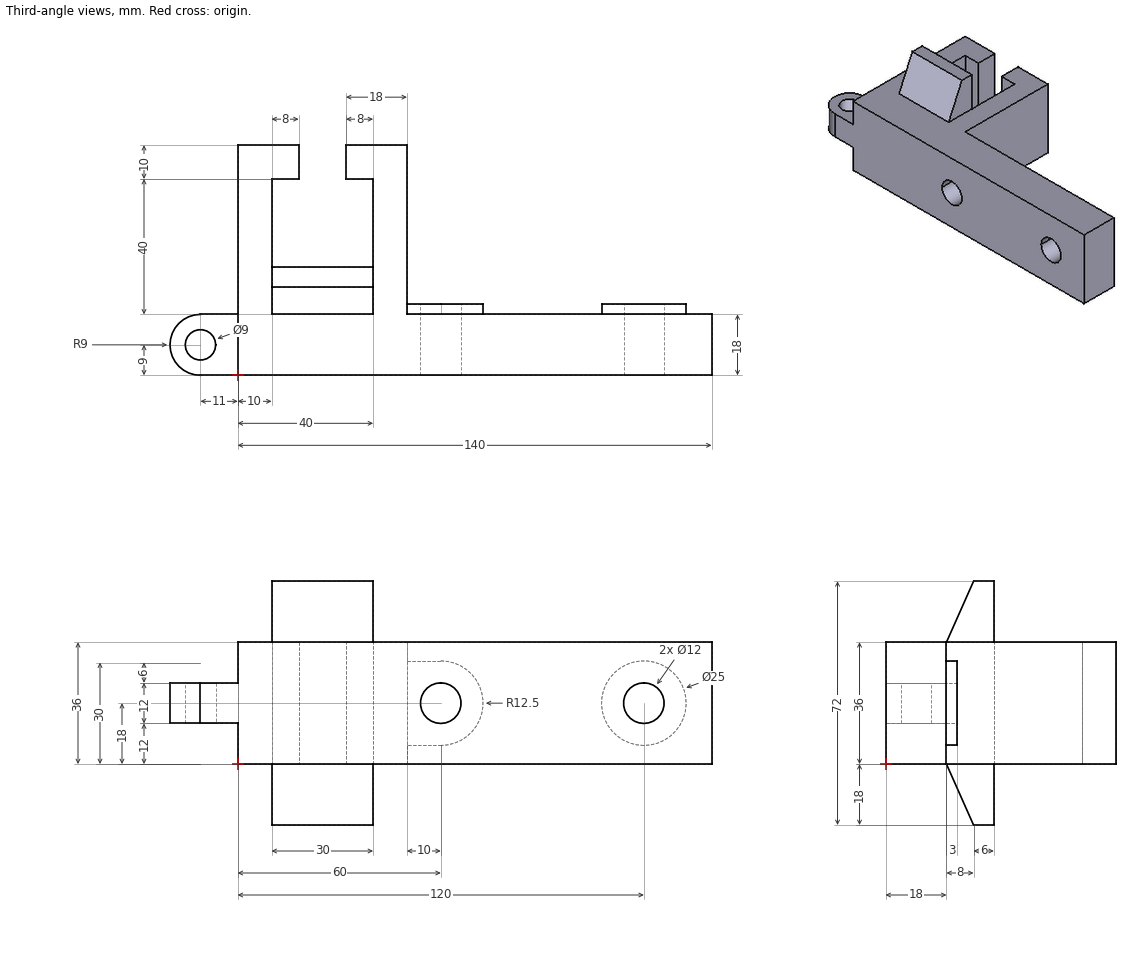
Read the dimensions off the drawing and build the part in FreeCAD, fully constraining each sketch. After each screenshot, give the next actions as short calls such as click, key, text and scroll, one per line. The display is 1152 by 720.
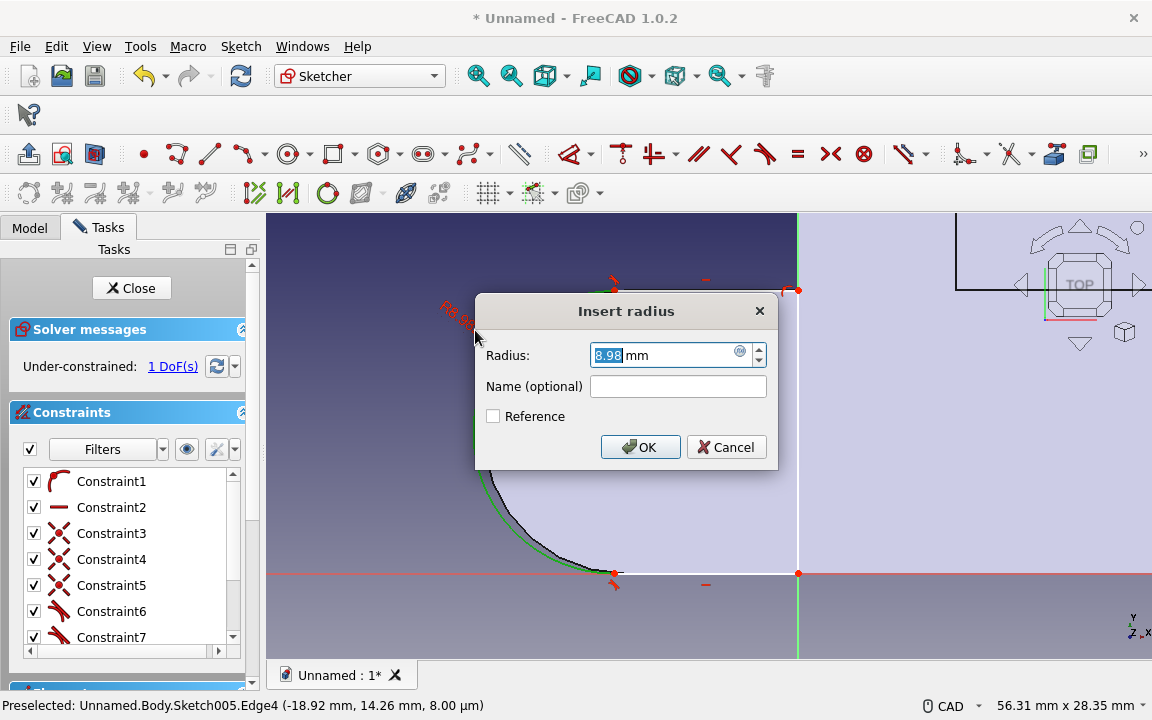
text(9)
key(Return)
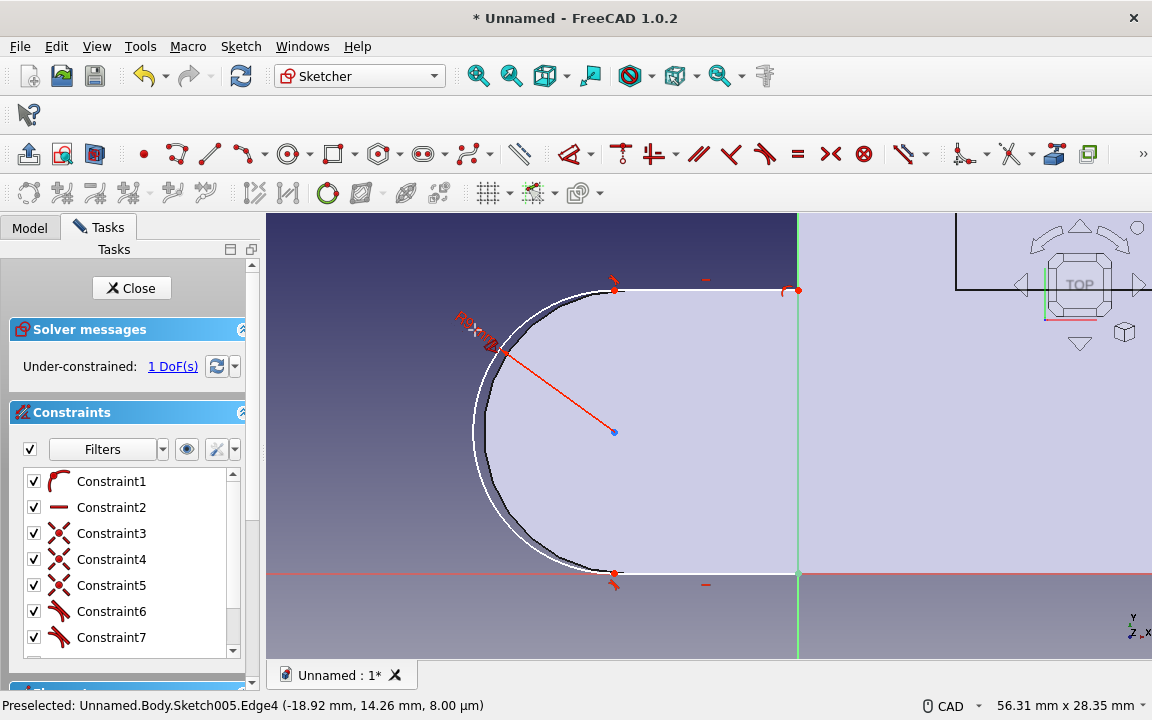
click(670, 290)
click(707, 256)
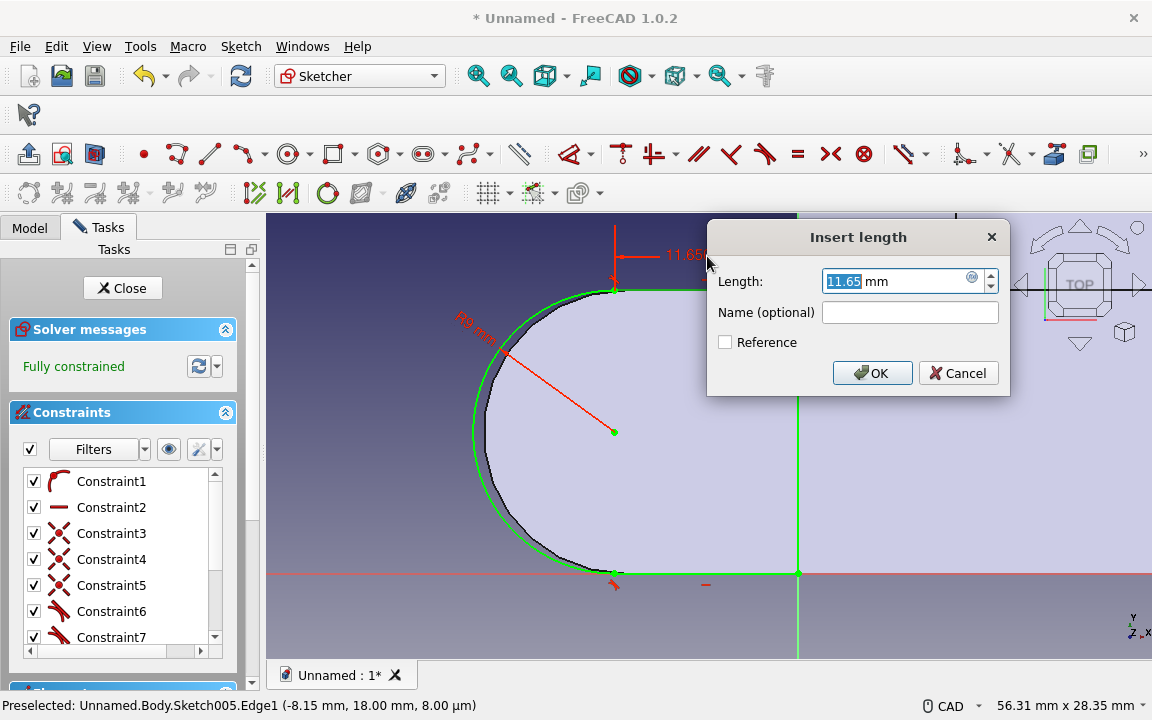
text(11)
key(Return)
key(Escape)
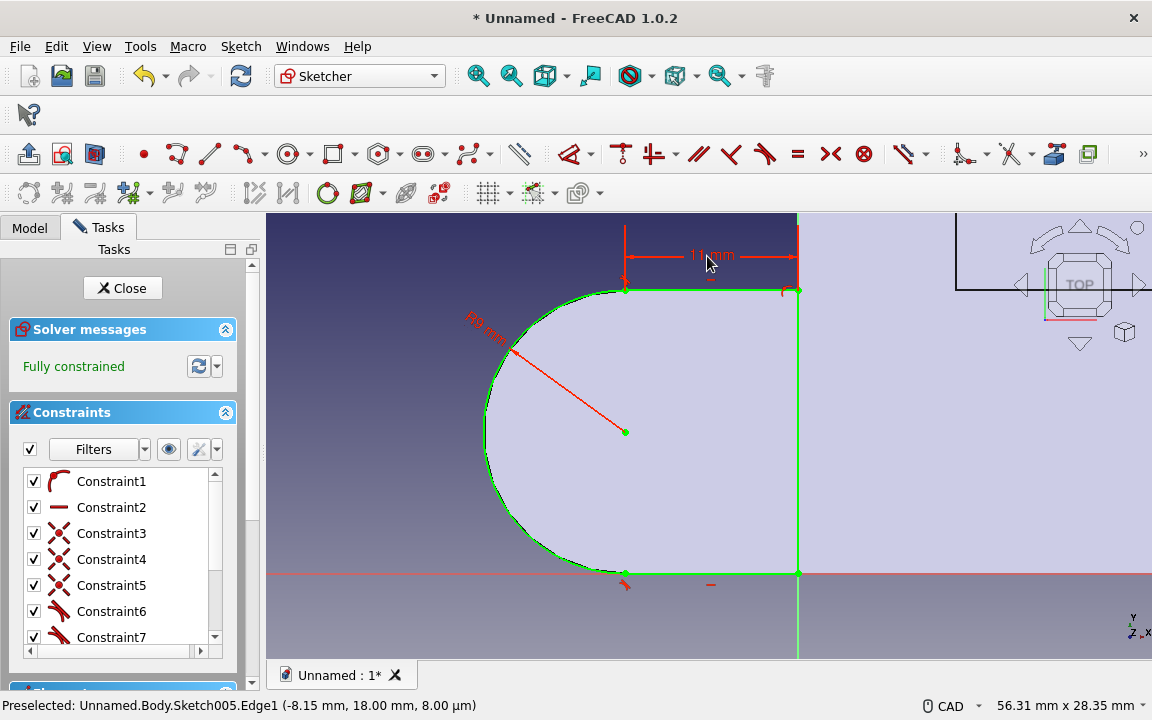
click(123, 288)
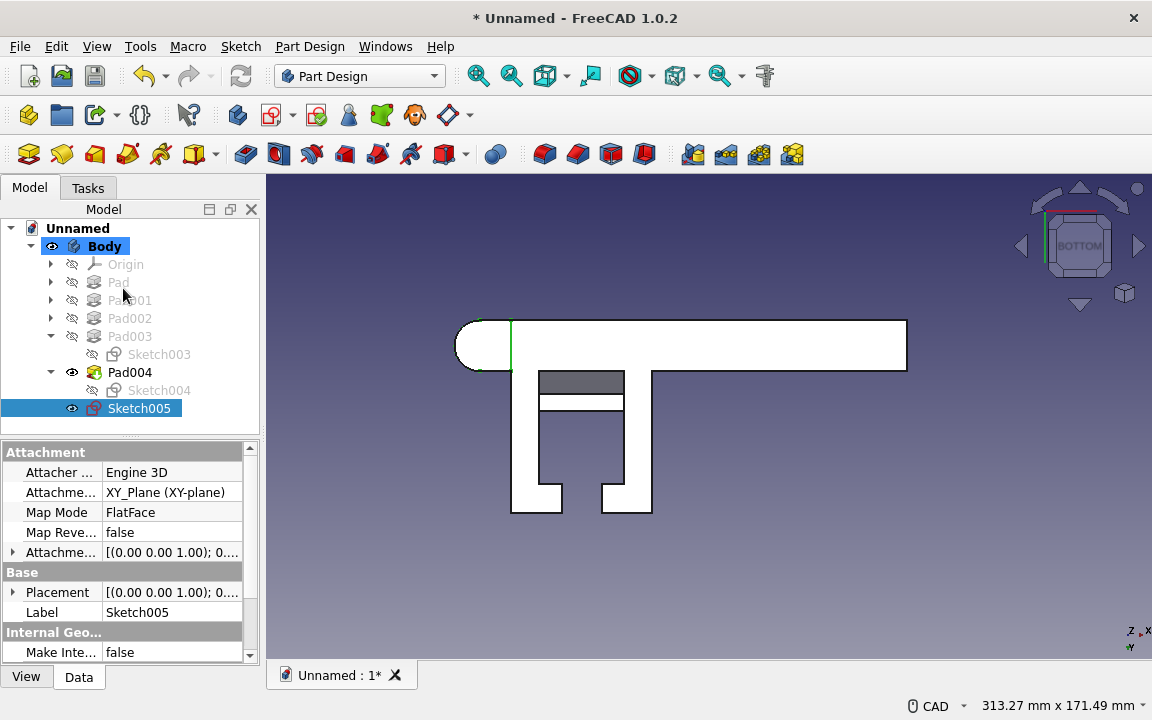
click(246, 154)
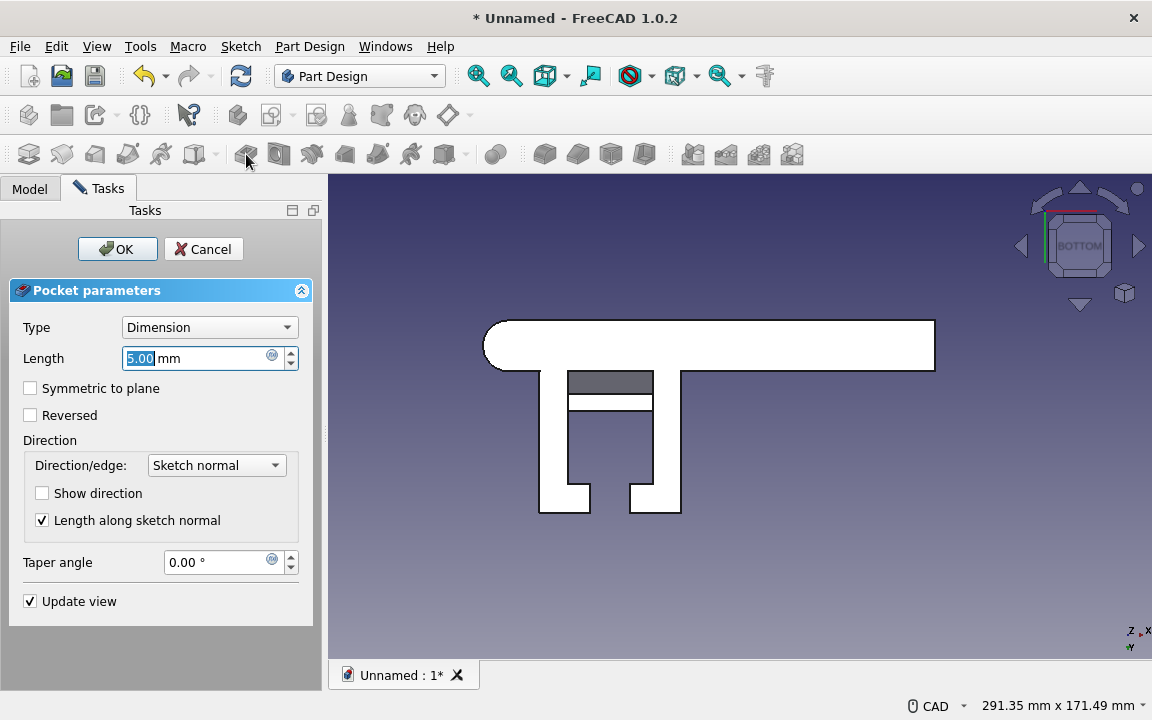
text(12)
key(Tab)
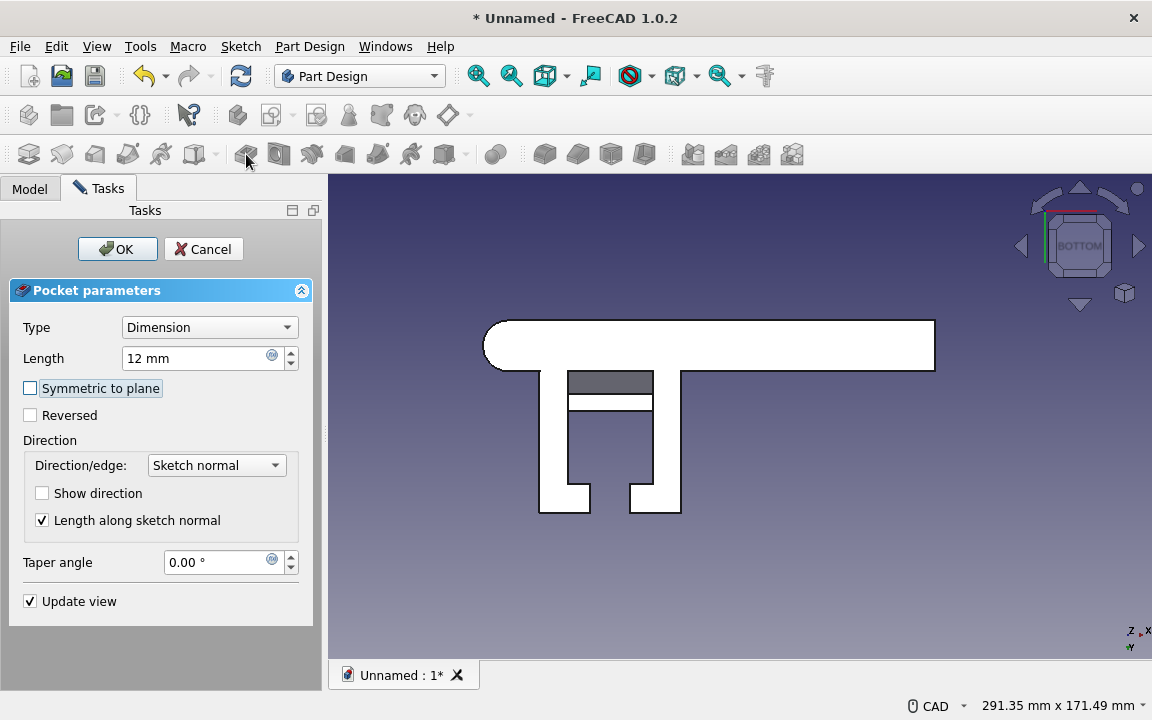
click(31, 415)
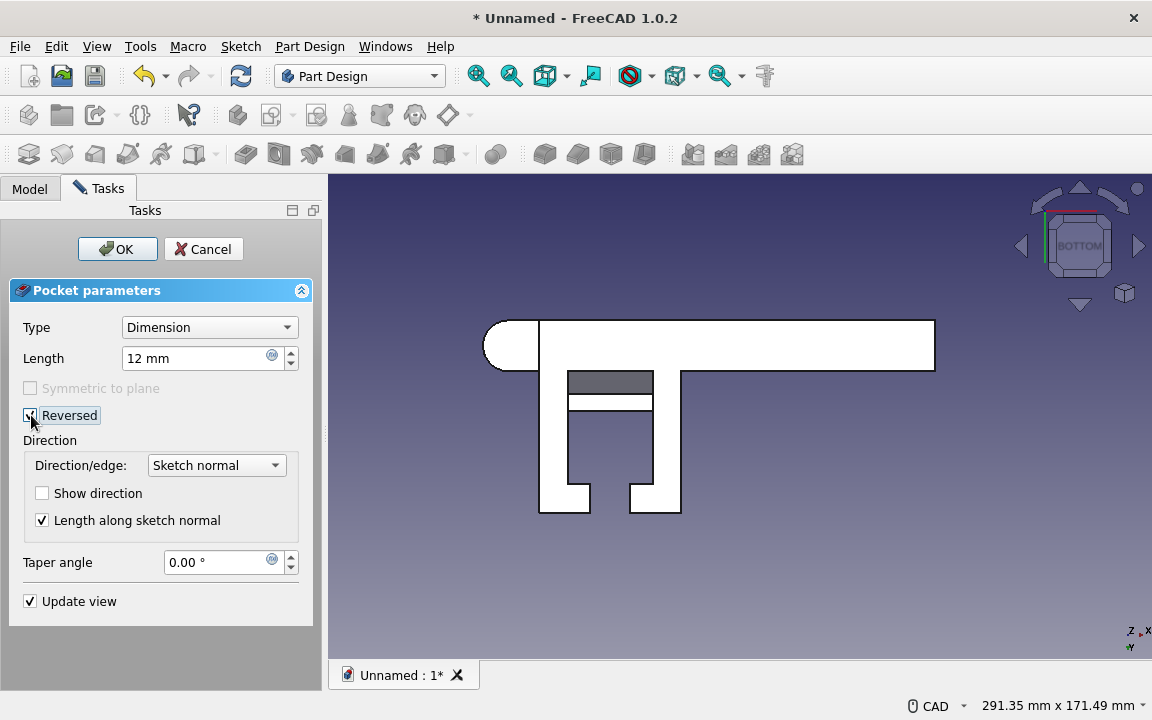
click(118, 249)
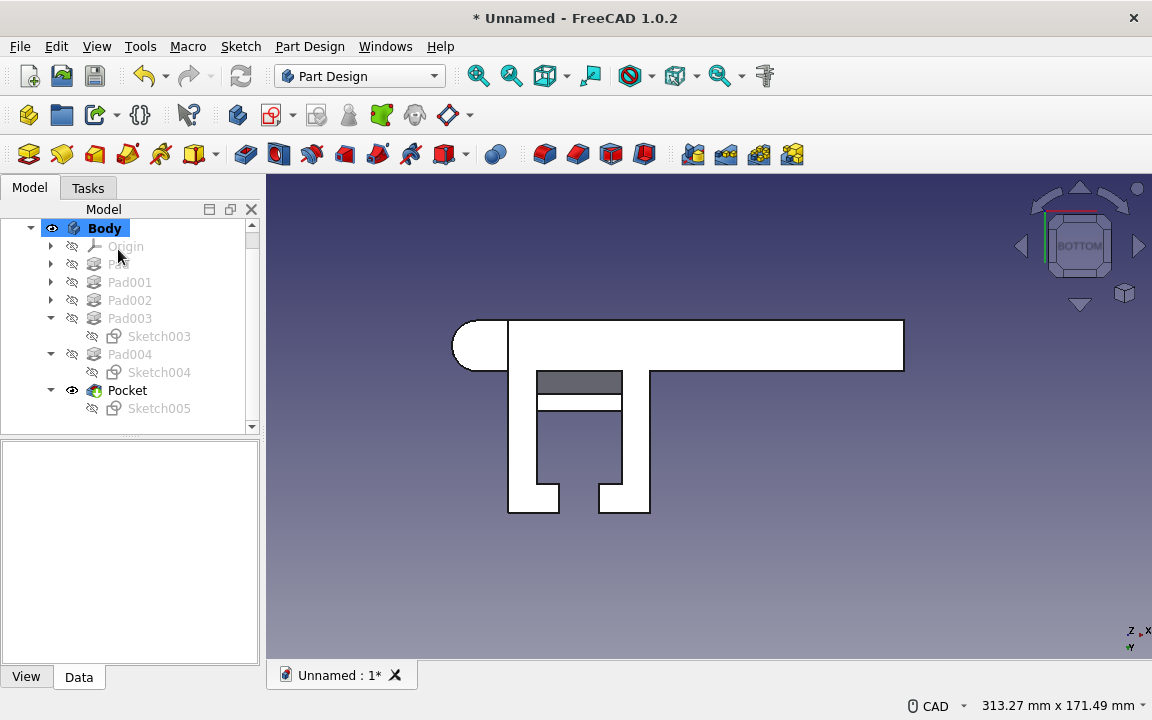
click(51, 246)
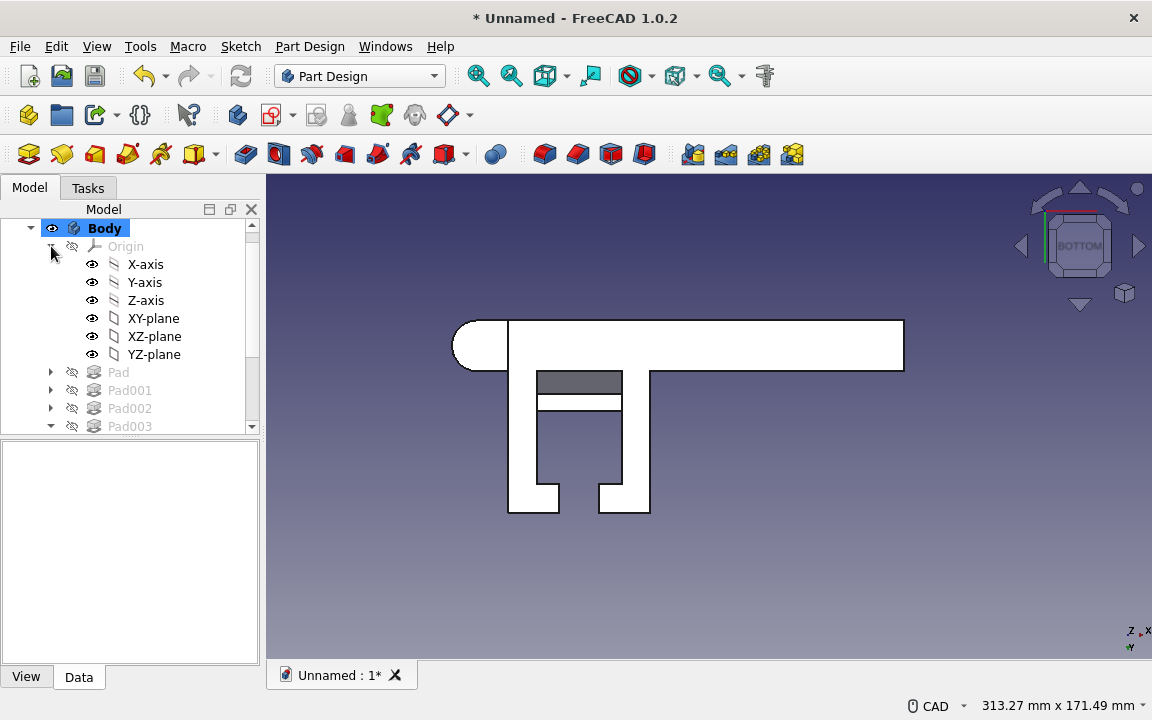
click(137, 318)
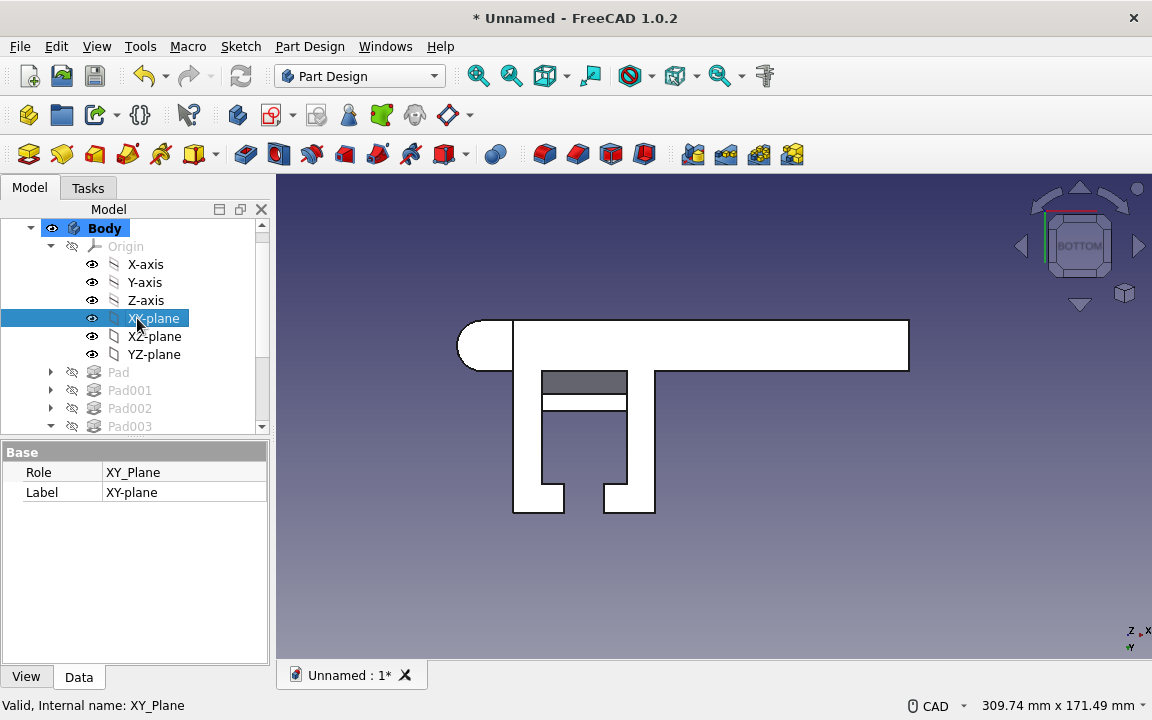
click(448, 116)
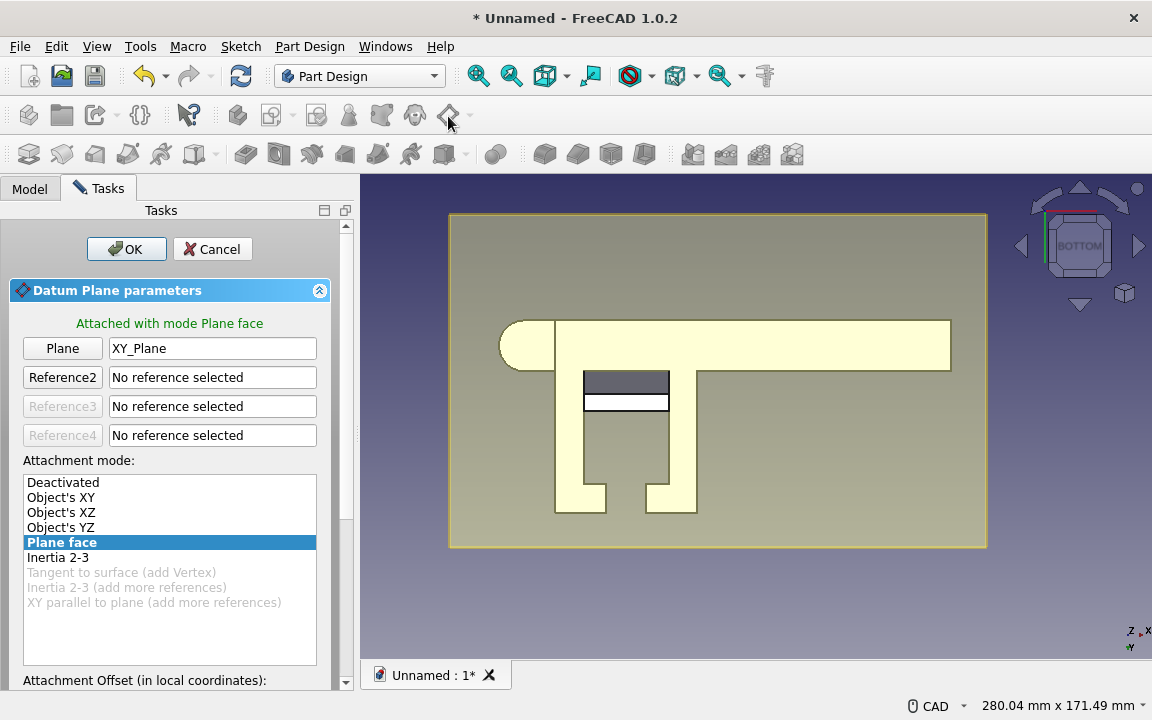
scroll(346, 455, down, 3)